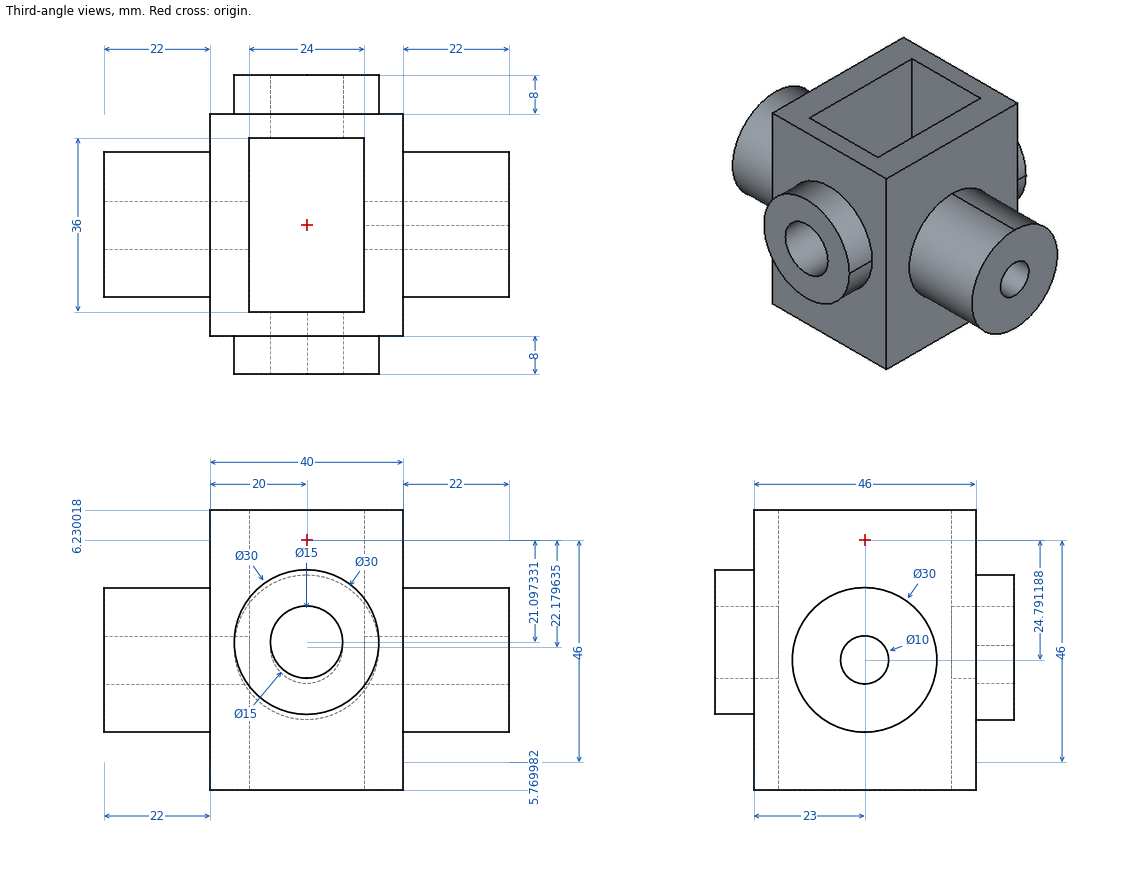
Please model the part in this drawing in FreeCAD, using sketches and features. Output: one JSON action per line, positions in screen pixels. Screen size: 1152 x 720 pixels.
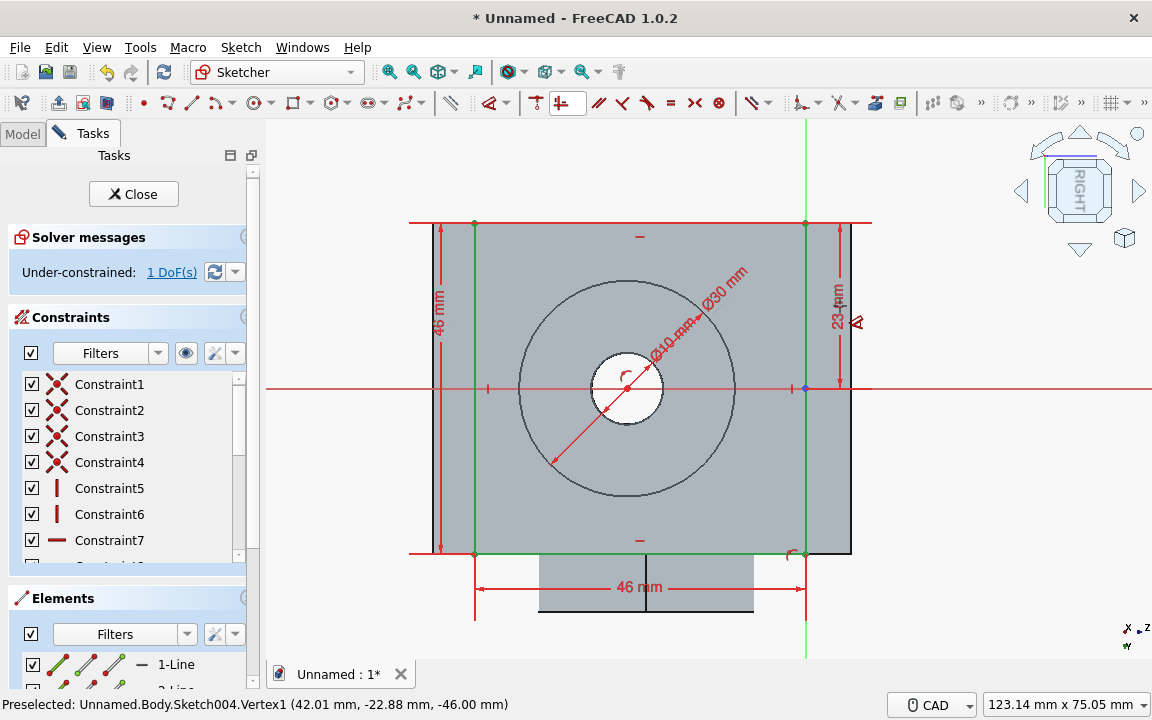
{"action": "left_click", "coordinate": [627, 389]}
{"action": "left_click", "coordinate": [675, 423]}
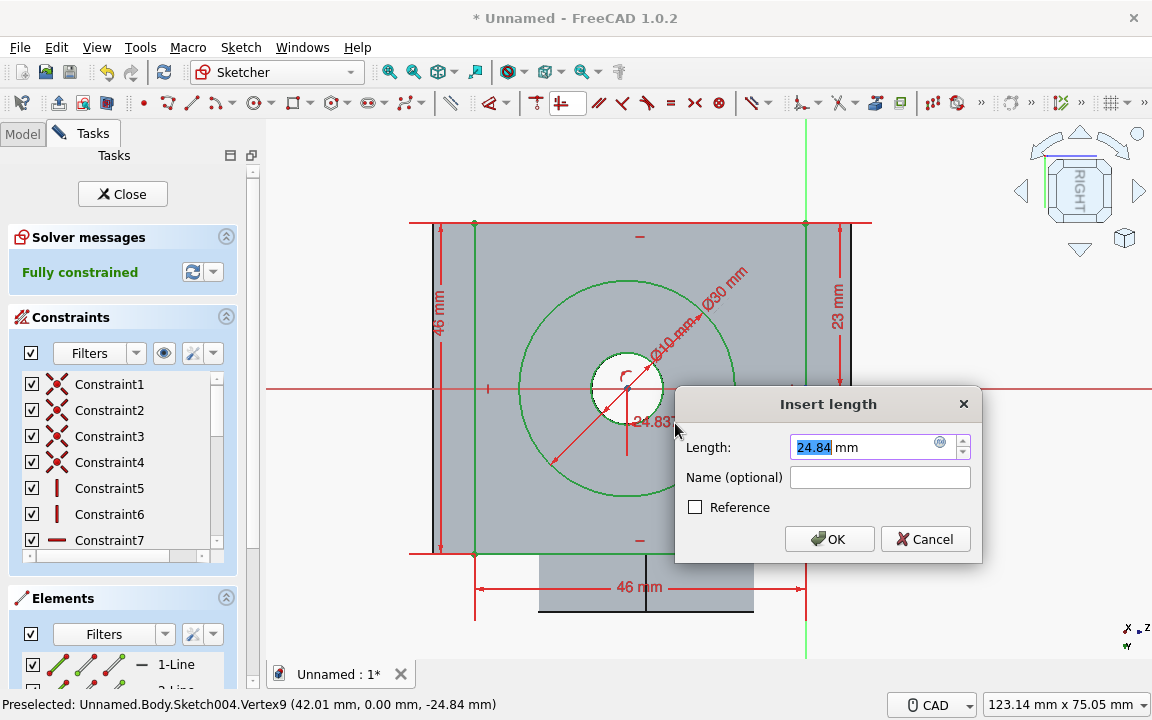
{"action": "type", "text": "24.791188"}
{"action": "key", "text": "Return"}
{"action": "key", "text": "Escape"}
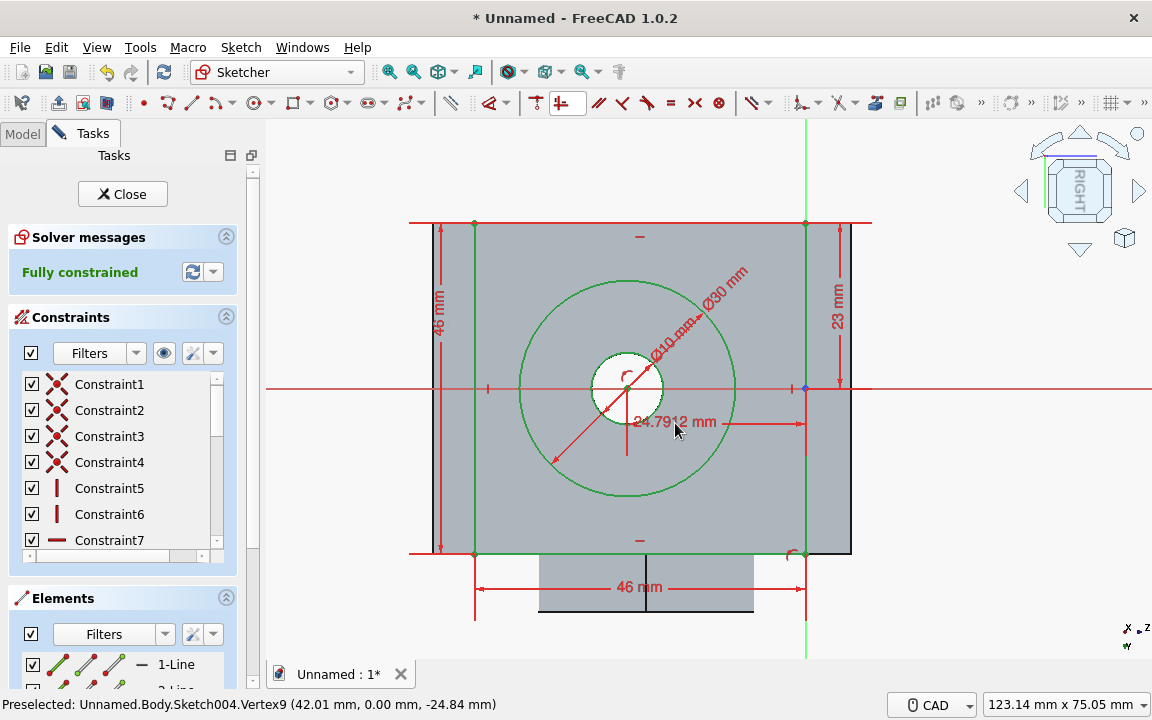
{"action": "left_click", "coordinate": [123, 194]}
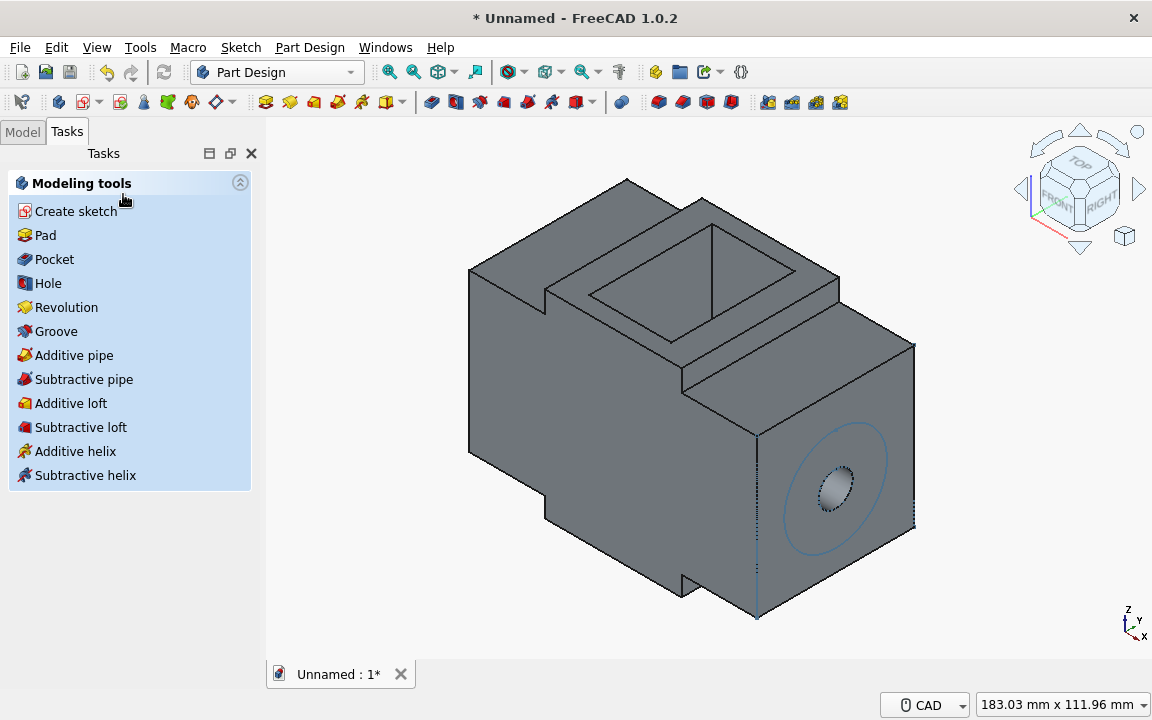
{"action": "left_click", "coordinate": [432, 102]}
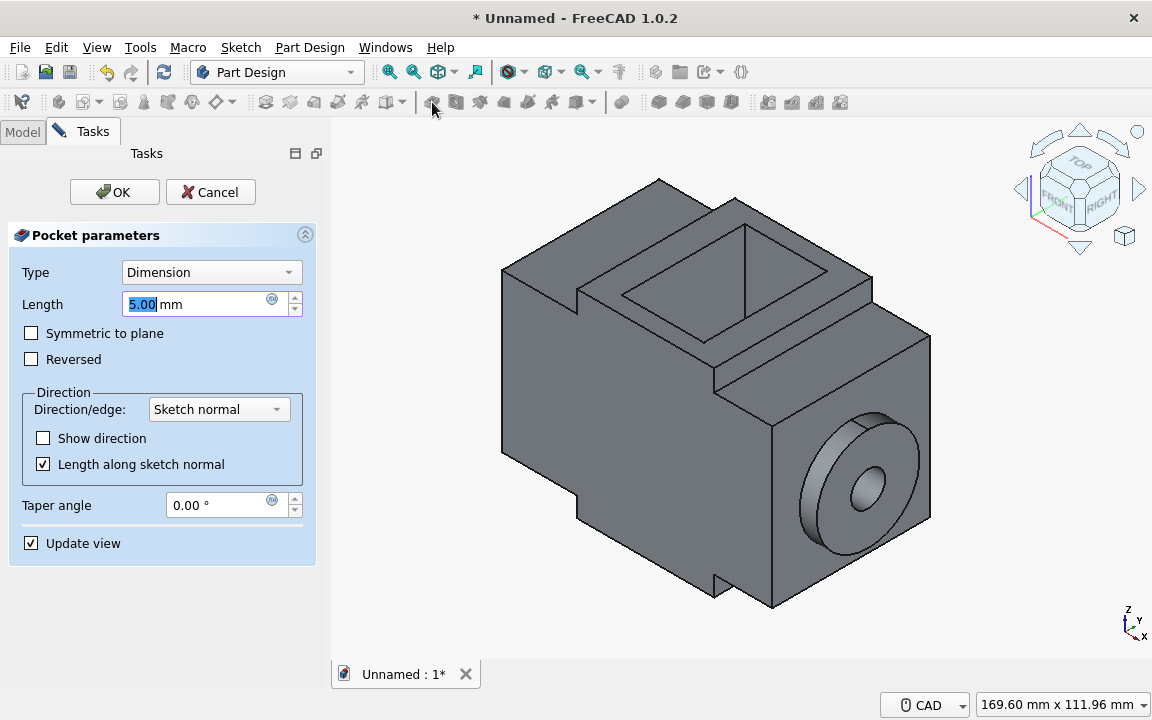
{"action": "type", "text": "22"}
{"action": "key", "text": "Tab"}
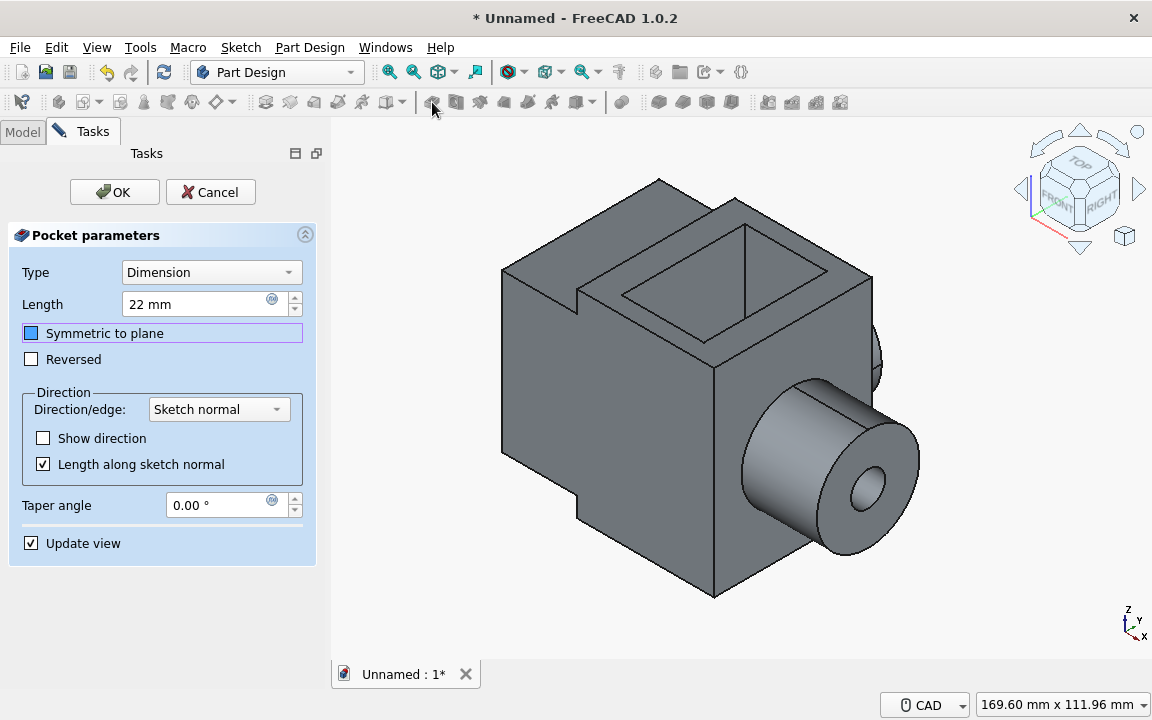
{"action": "left_click", "coordinate": [115, 192]}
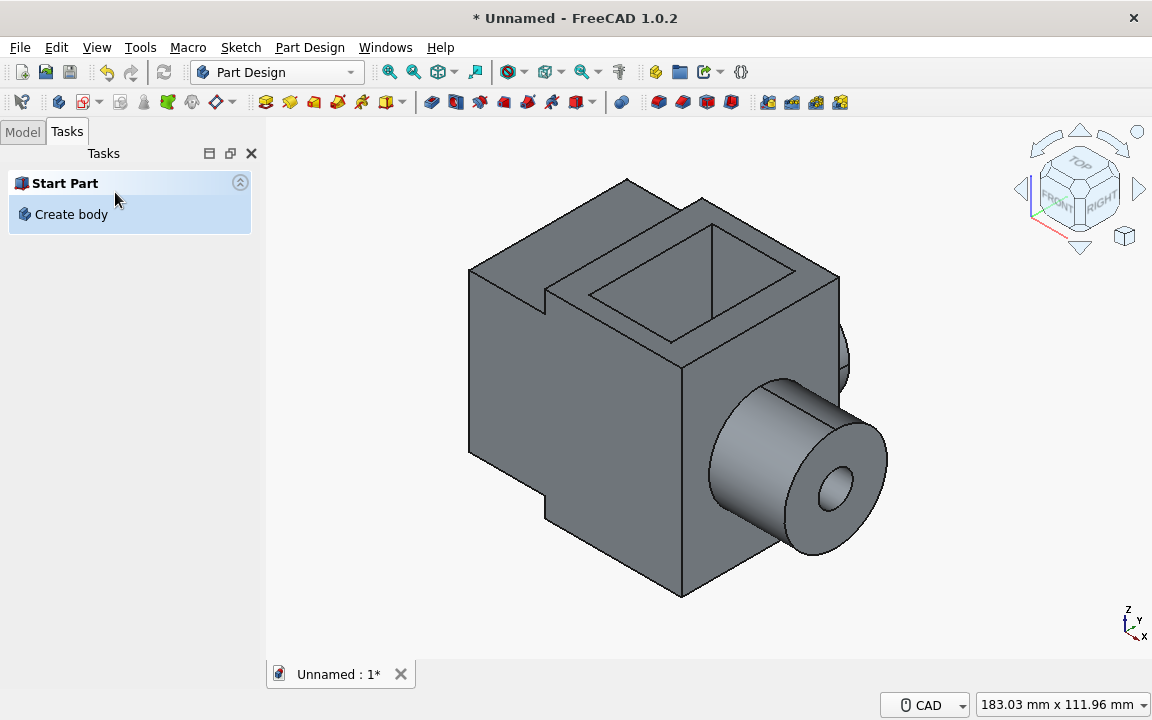
{"action": "key", "text": "6"}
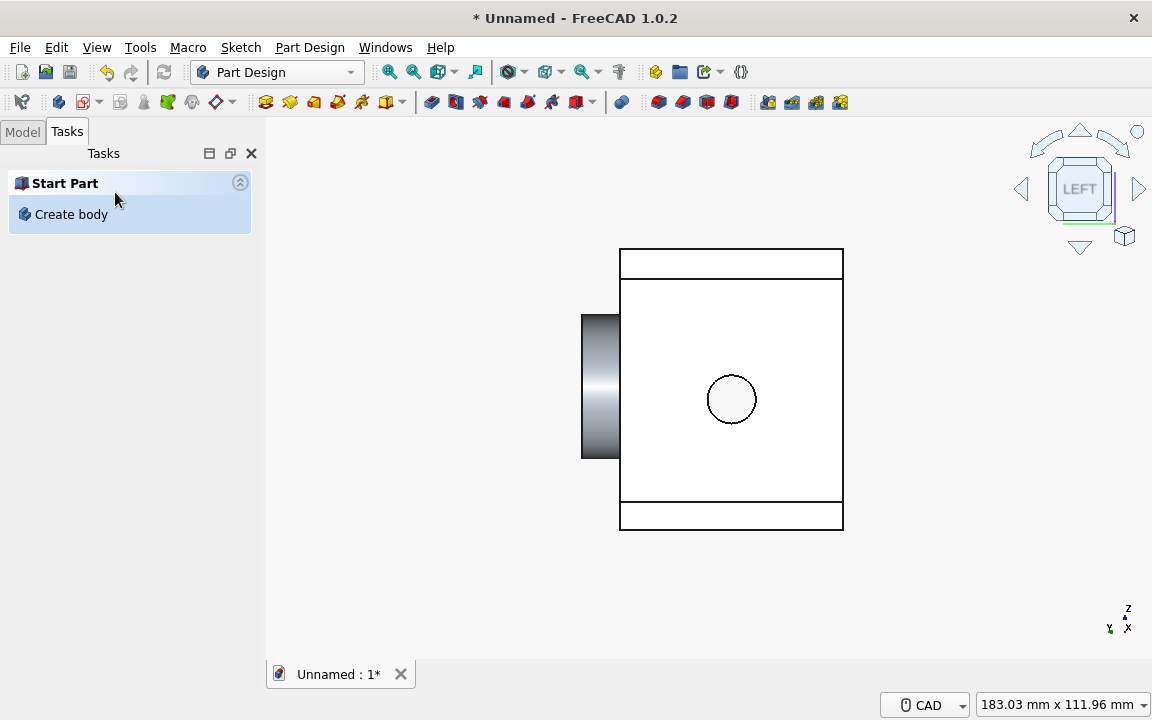
{"action": "left_click", "coordinate": [636, 263]}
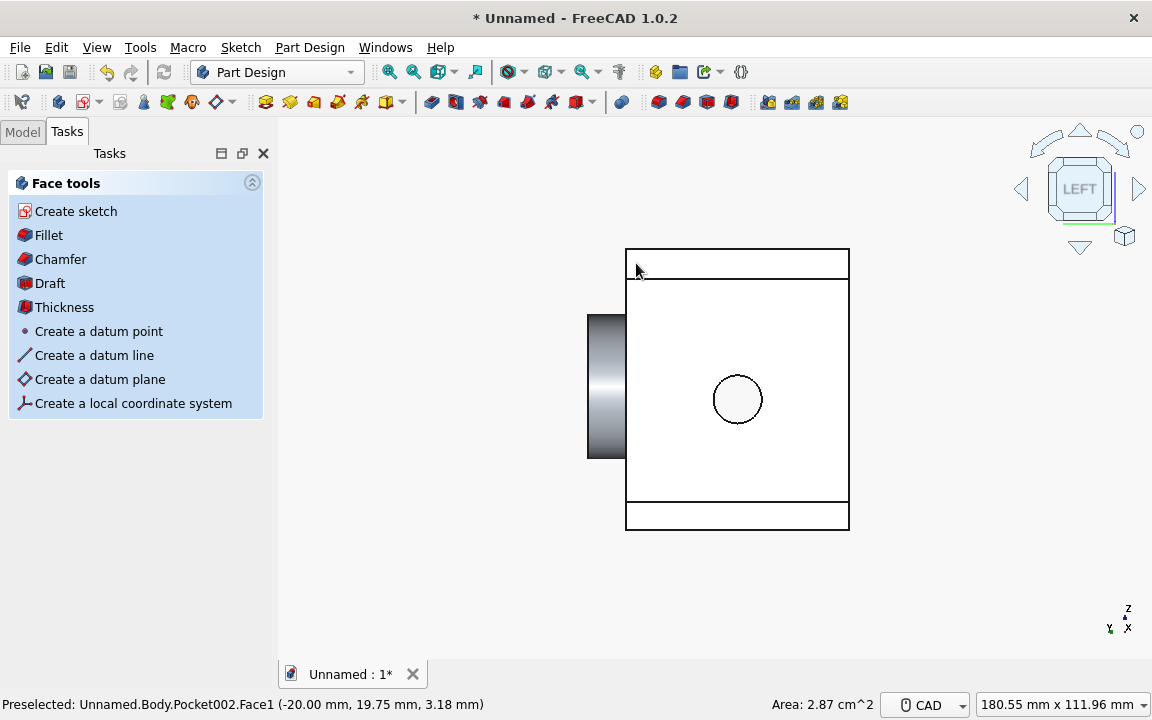
{"action": "left_click", "coordinate": [84, 102]}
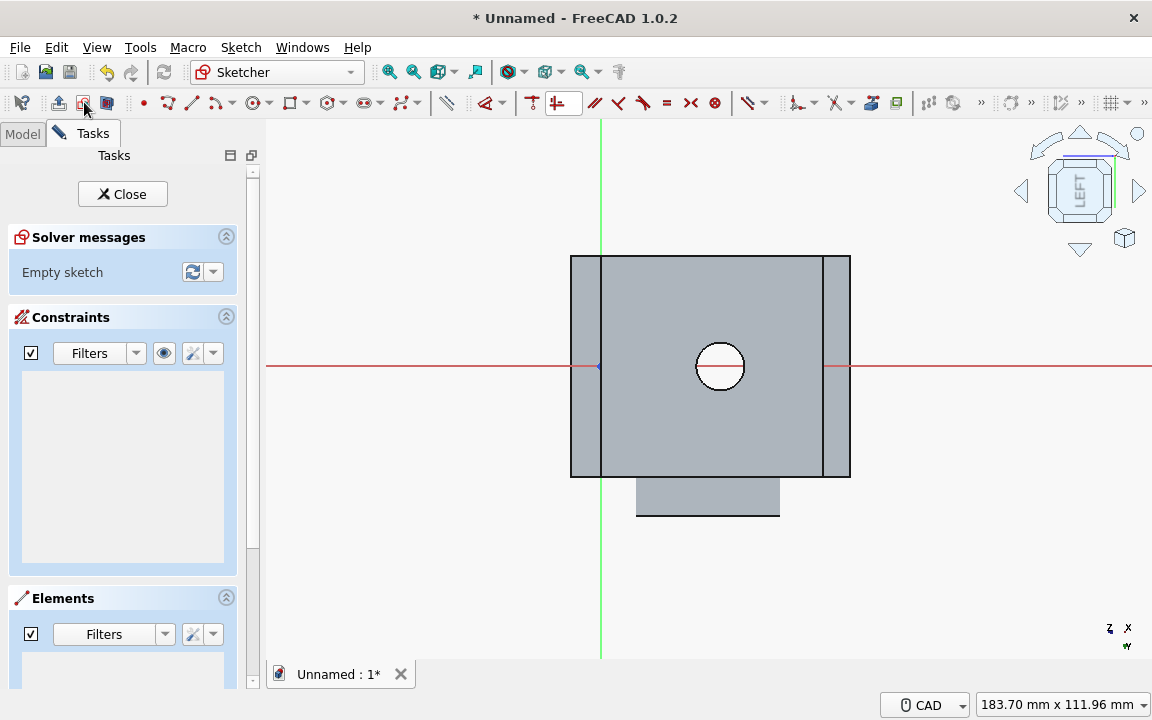
{"action": "left_click", "coordinate": [108, 104]}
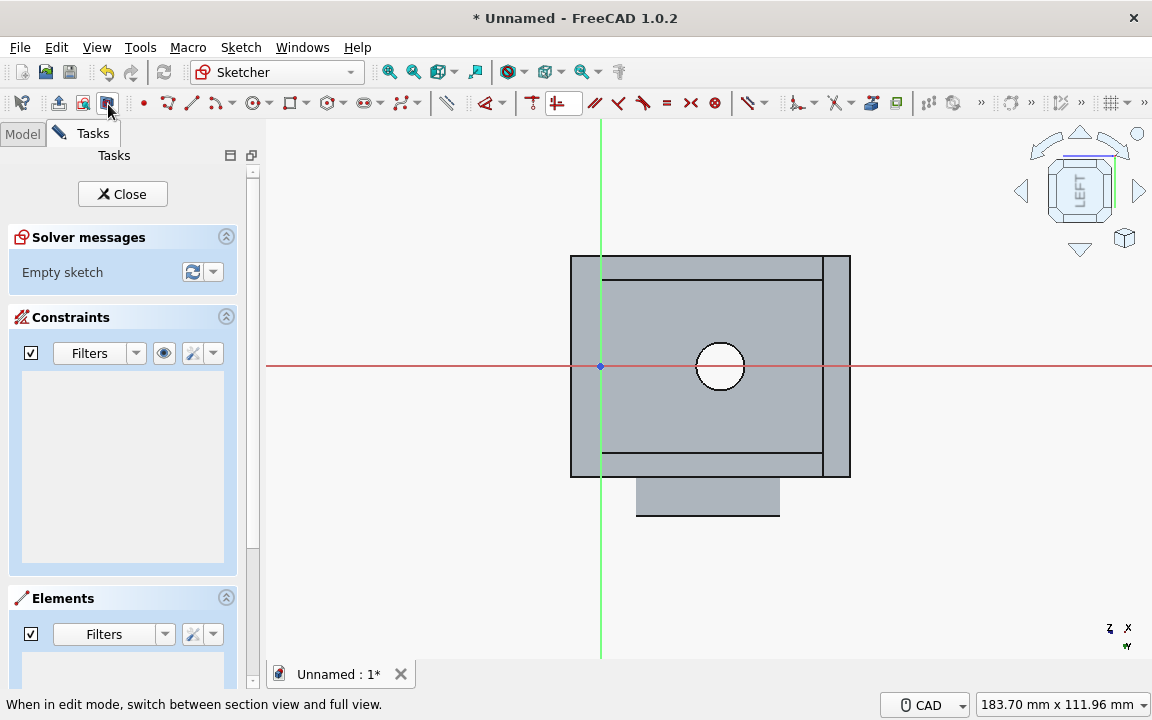
{"action": "scroll", "coordinate": [856, 321], "scroll_direction": "up", "scroll_amount": 2}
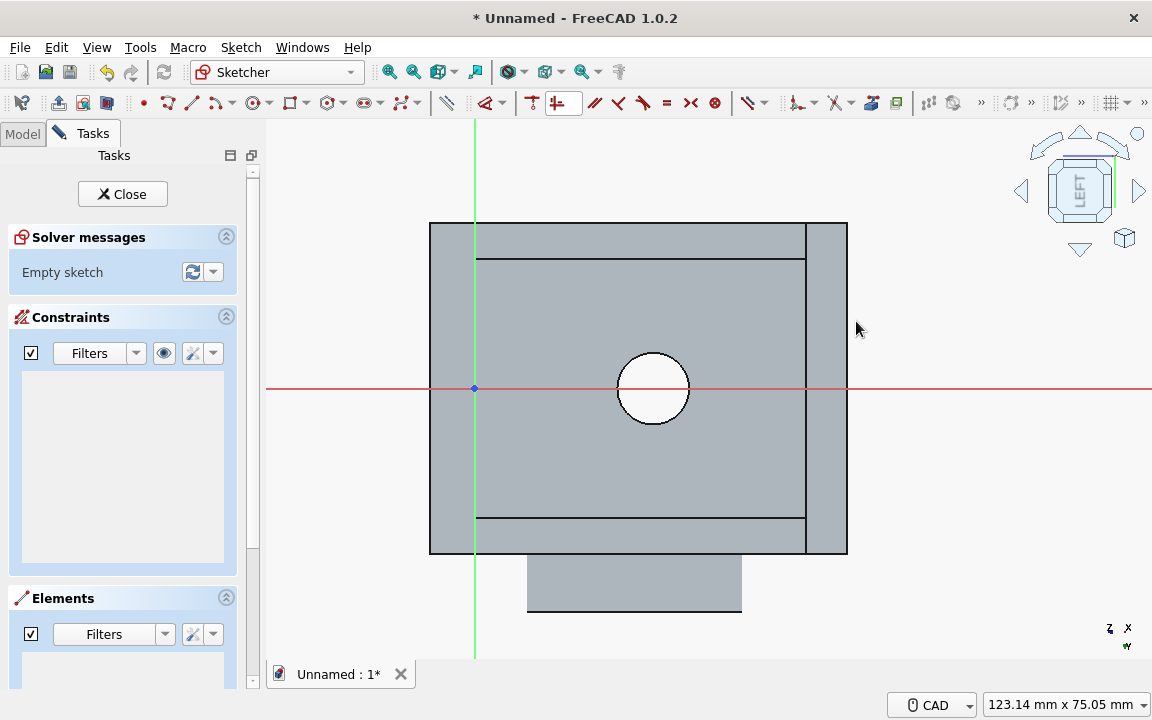
{"action": "left_click", "coordinate": [290, 104]}